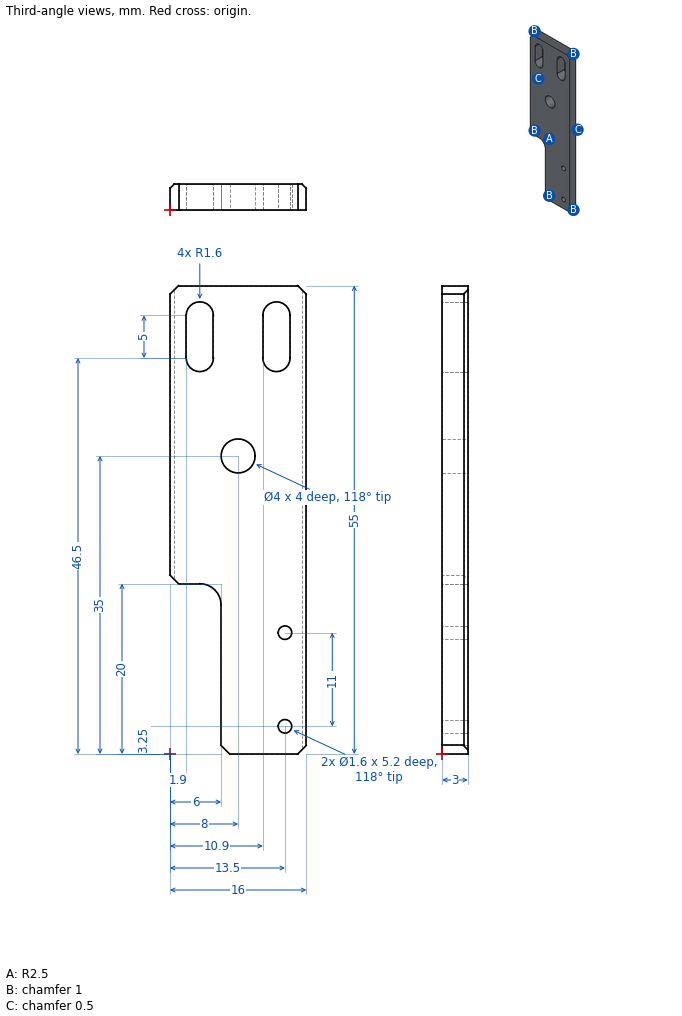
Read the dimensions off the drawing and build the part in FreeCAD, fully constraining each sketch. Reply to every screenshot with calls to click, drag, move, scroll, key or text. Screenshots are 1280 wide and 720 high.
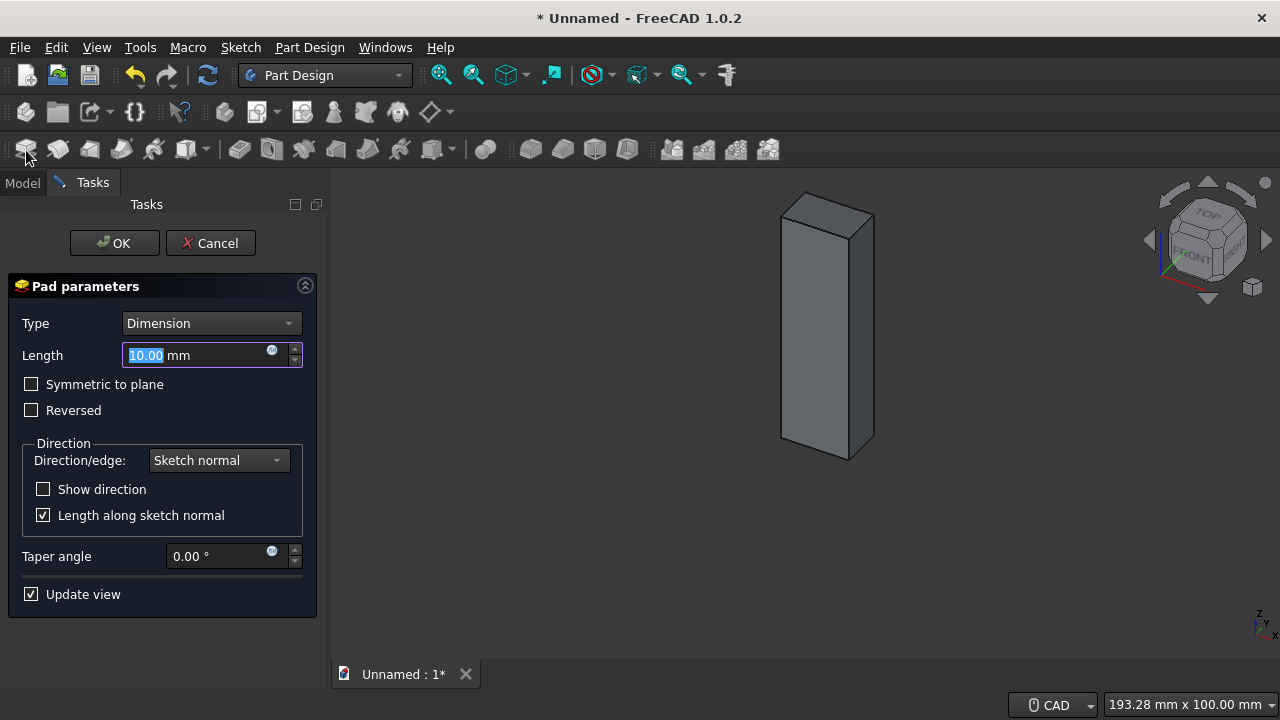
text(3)
key(Tab)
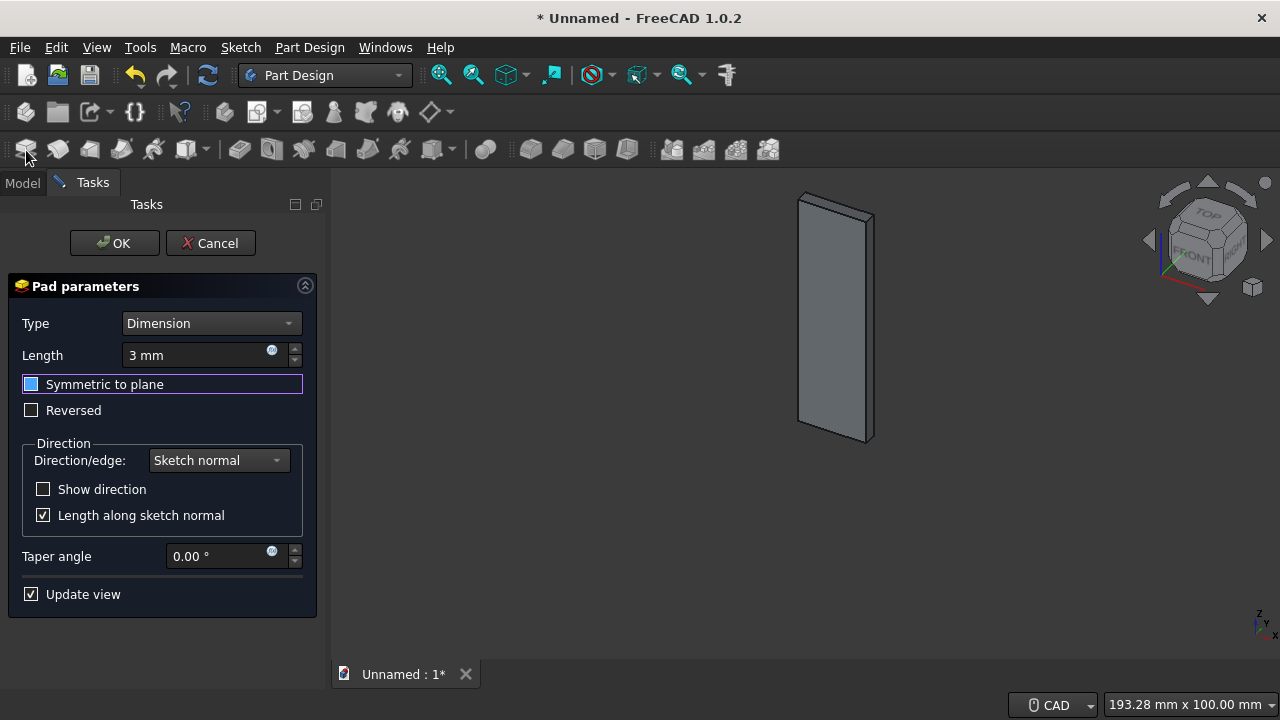
click(30, 410)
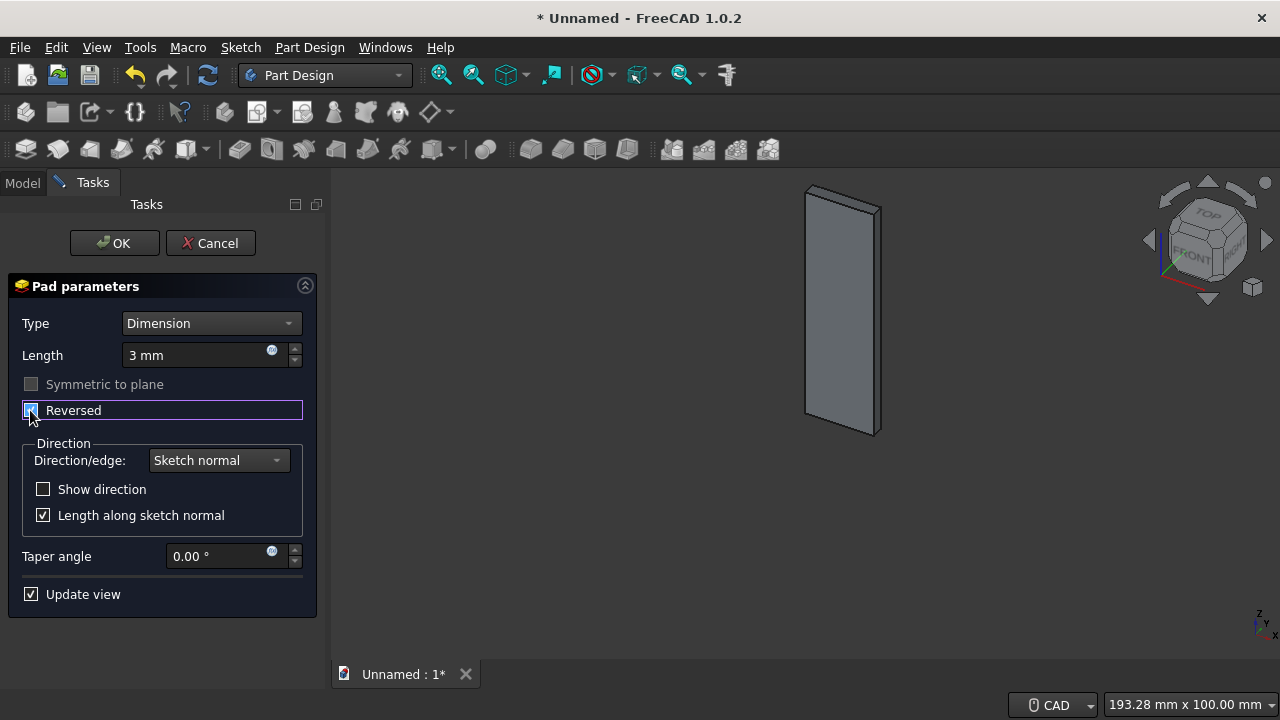
click(115, 243)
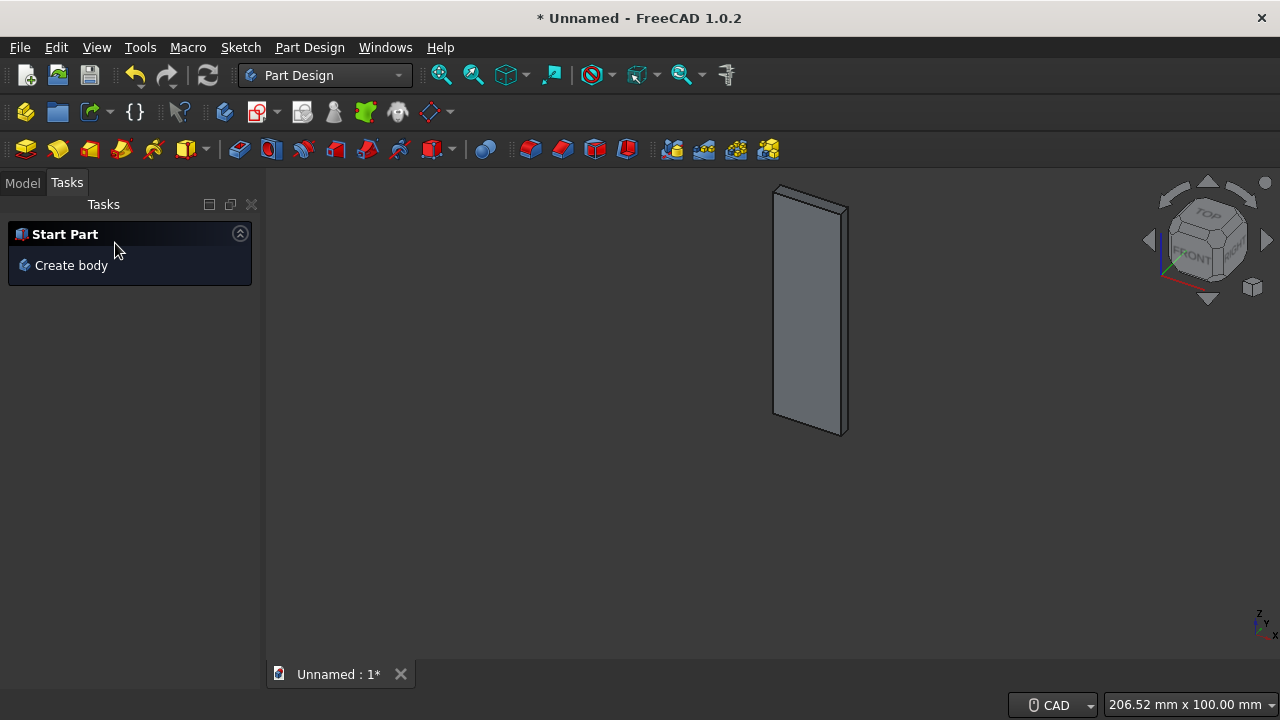
click(258, 112)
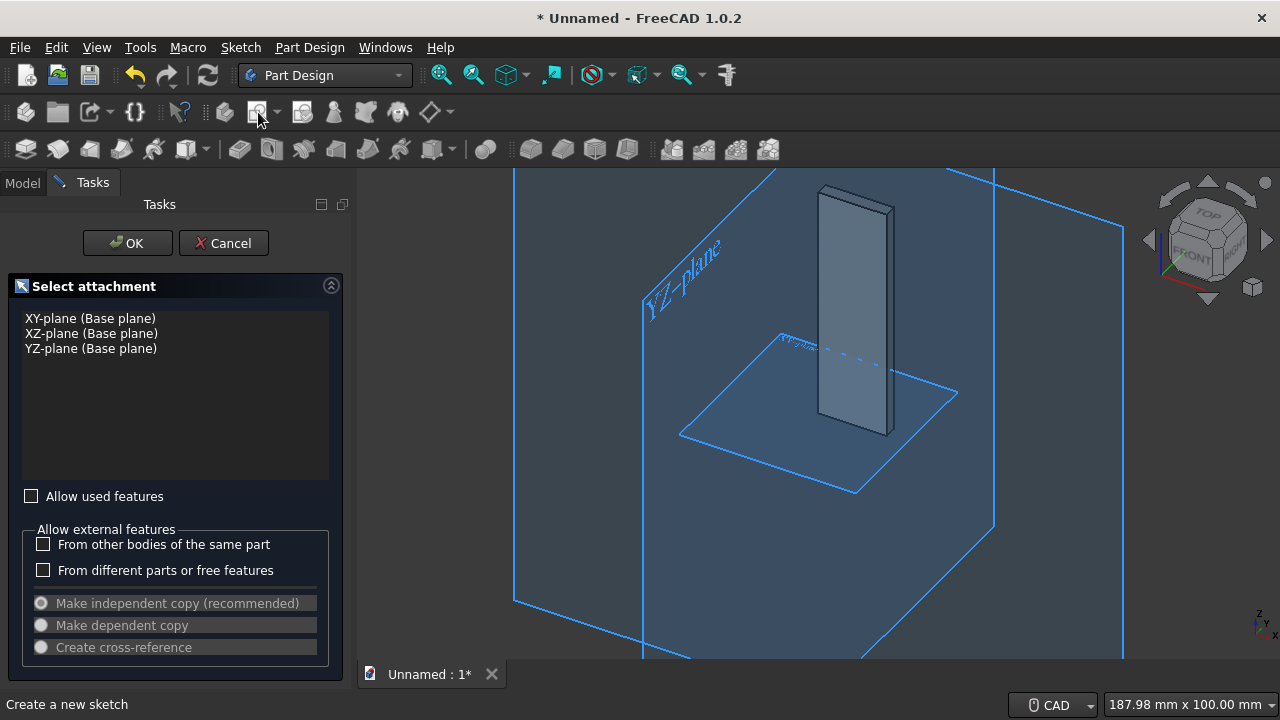
click(82, 334)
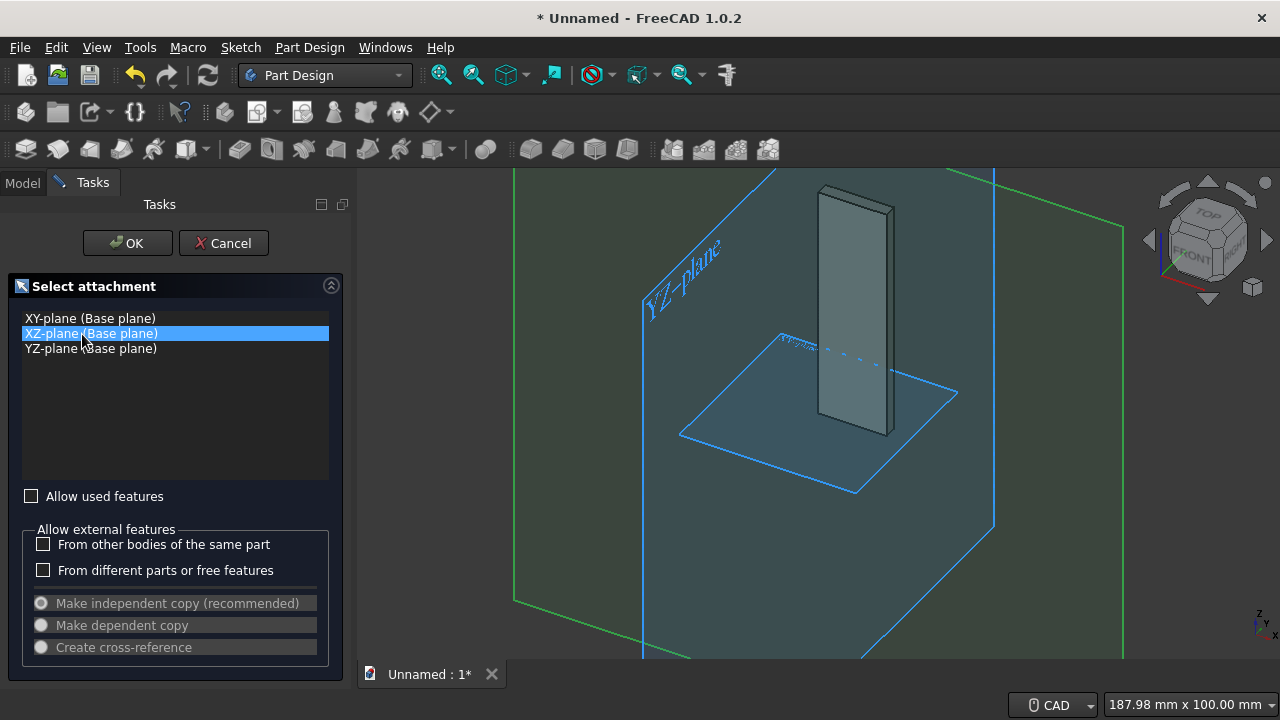
click(128, 243)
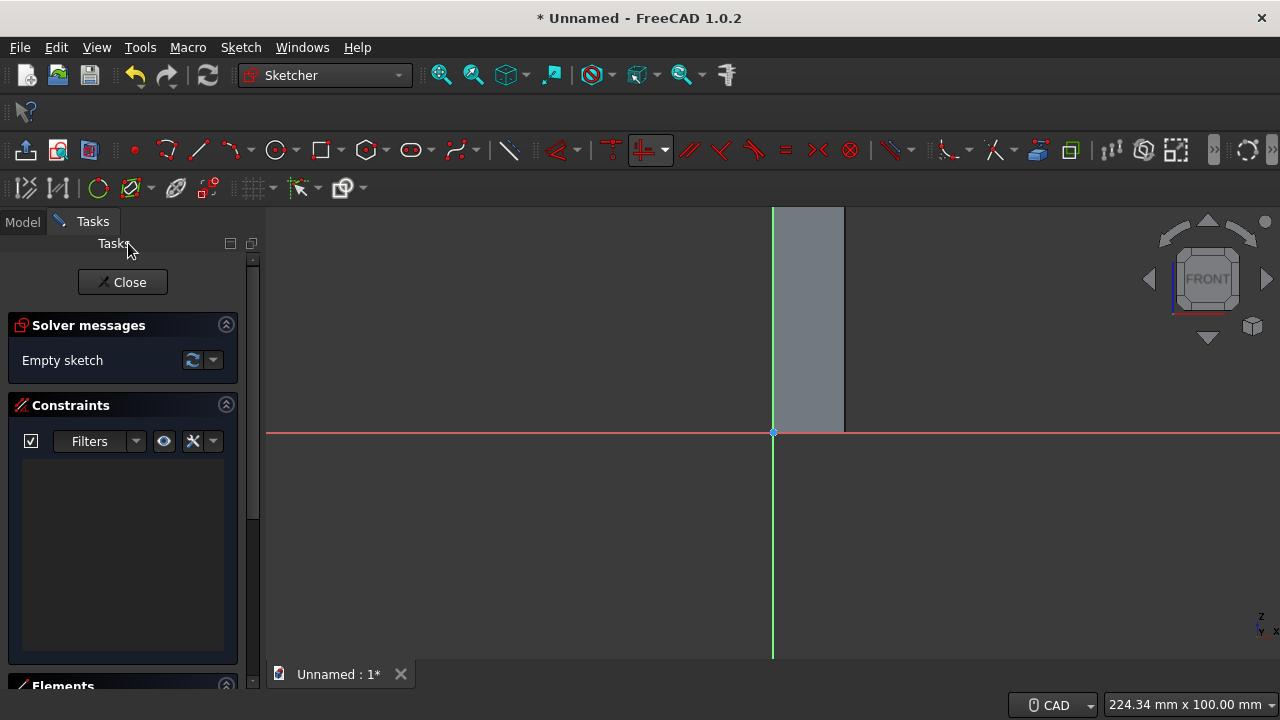
scroll(704, 433, down, 5)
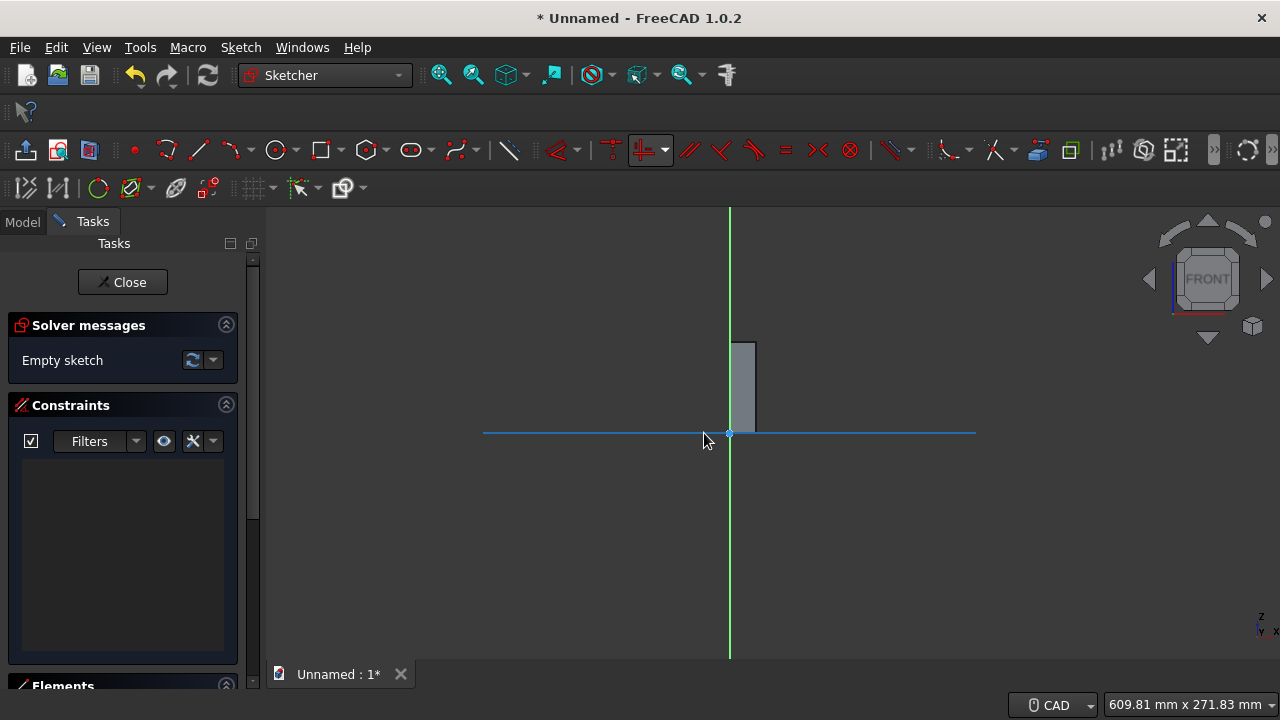
scroll(745, 348, up, 15)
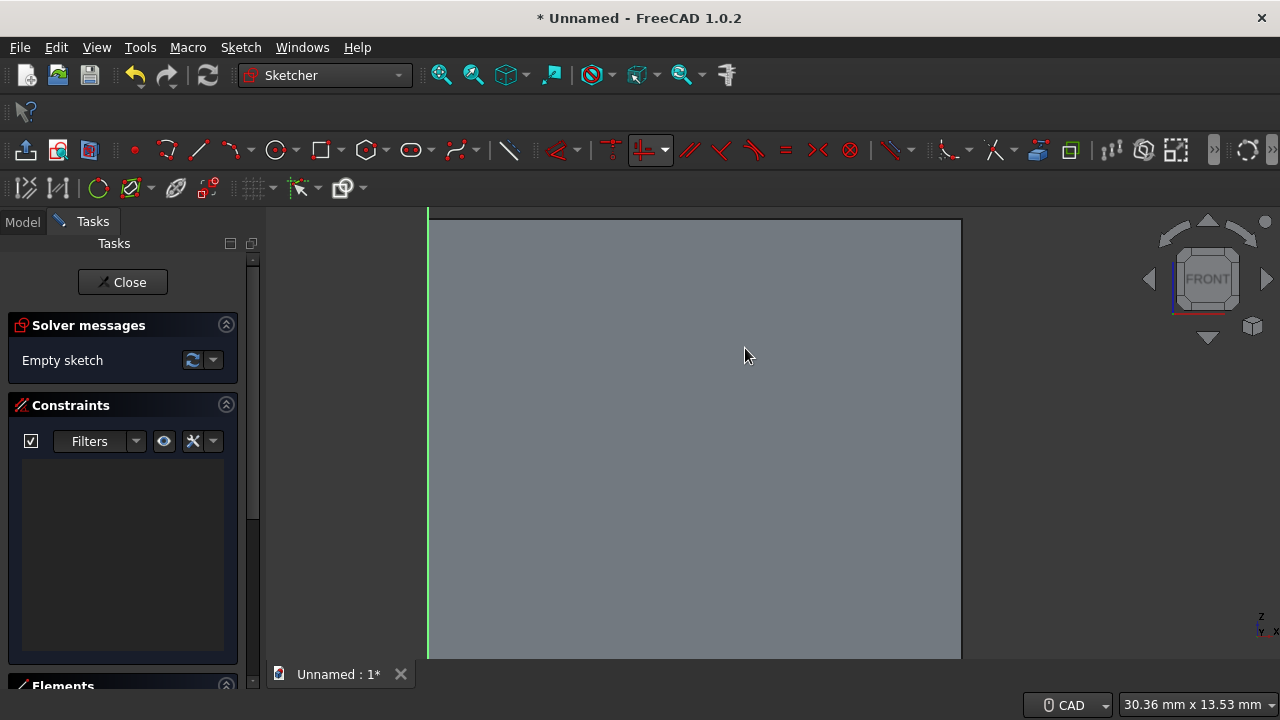
click(412, 150)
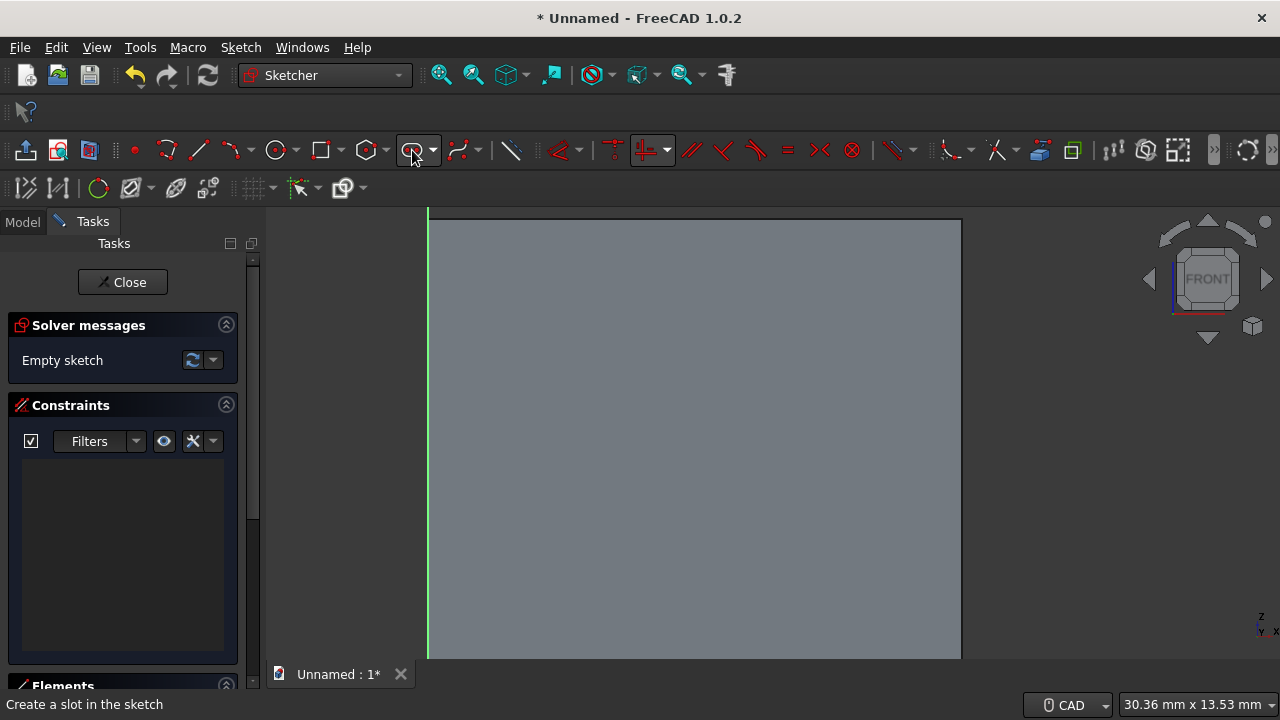
click(545, 503)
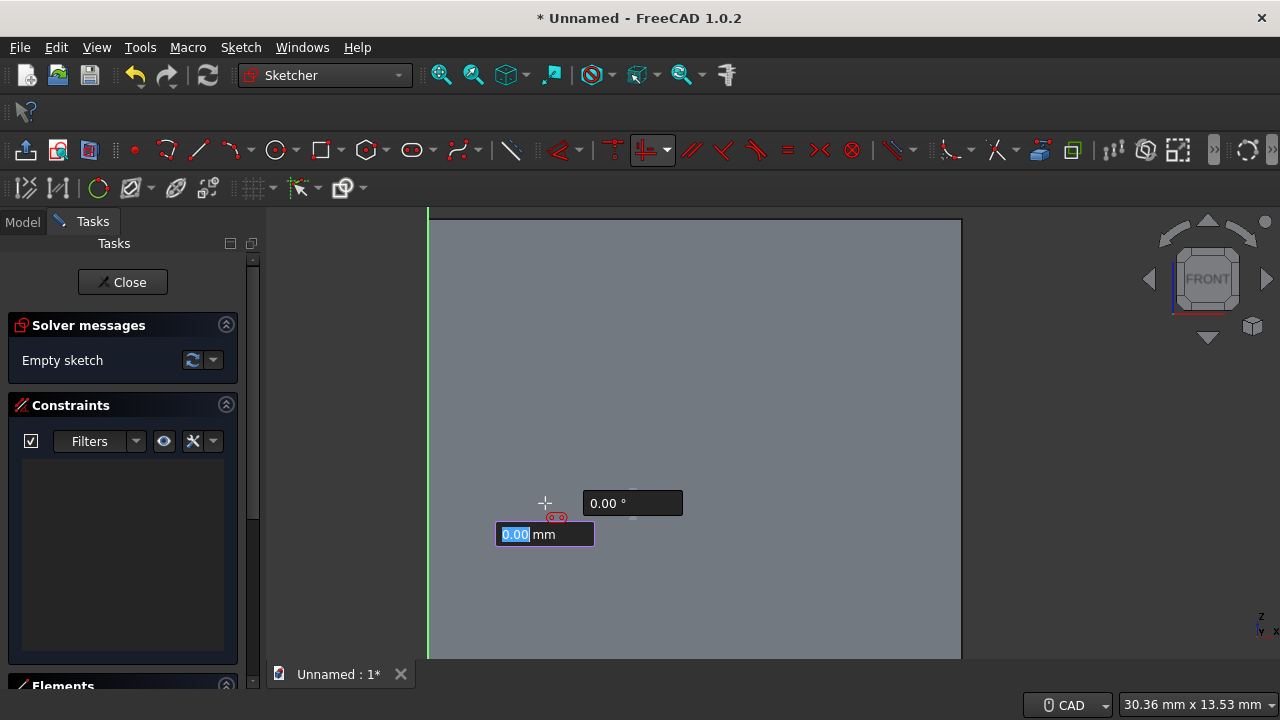
click(545, 336)